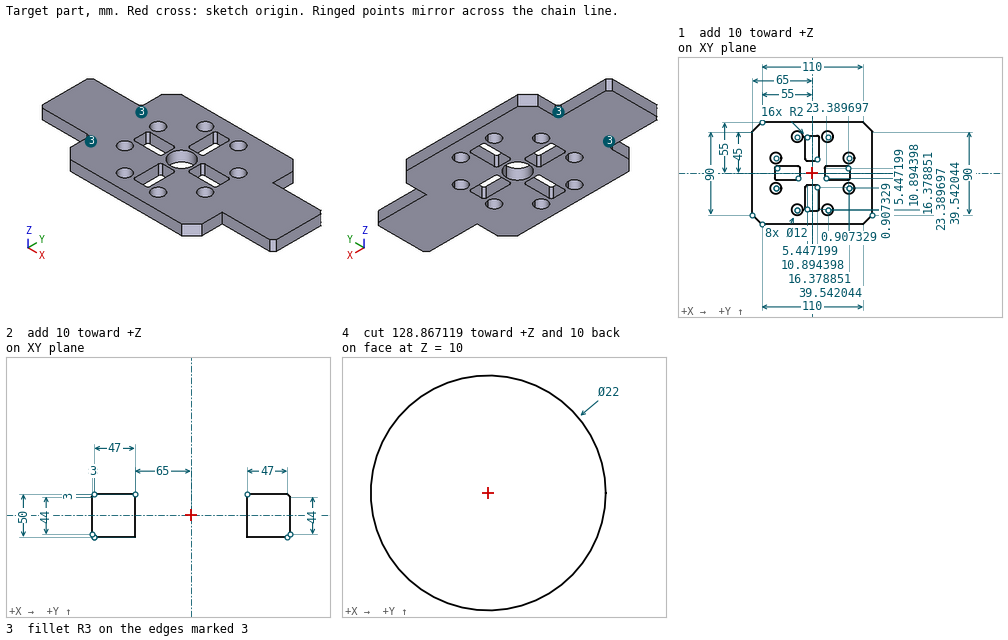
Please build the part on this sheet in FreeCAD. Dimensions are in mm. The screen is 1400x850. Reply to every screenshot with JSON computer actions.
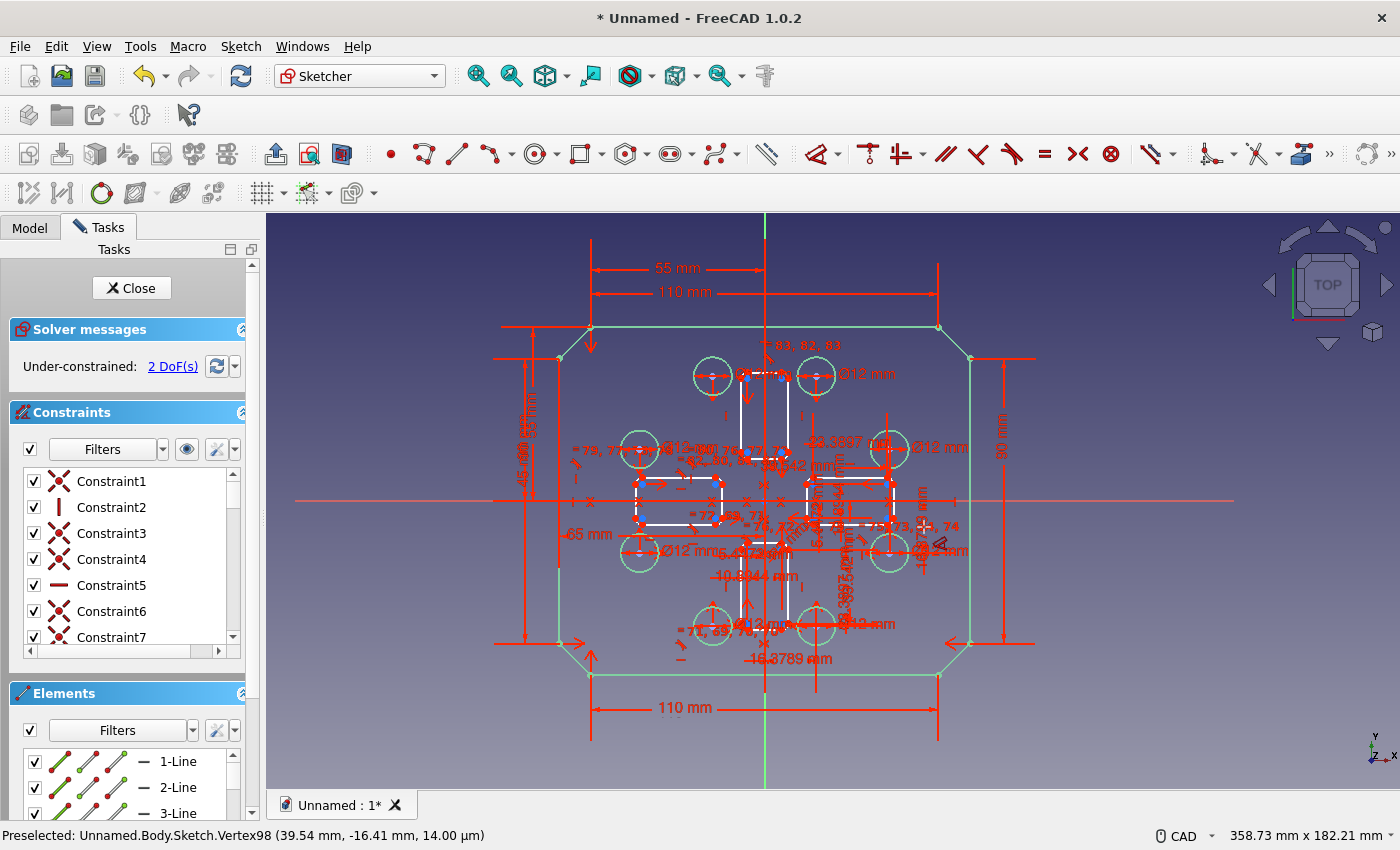
{"action": "scroll", "coordinate": [788, 624], "scroll_direction": "up", "scroll_amount": 14}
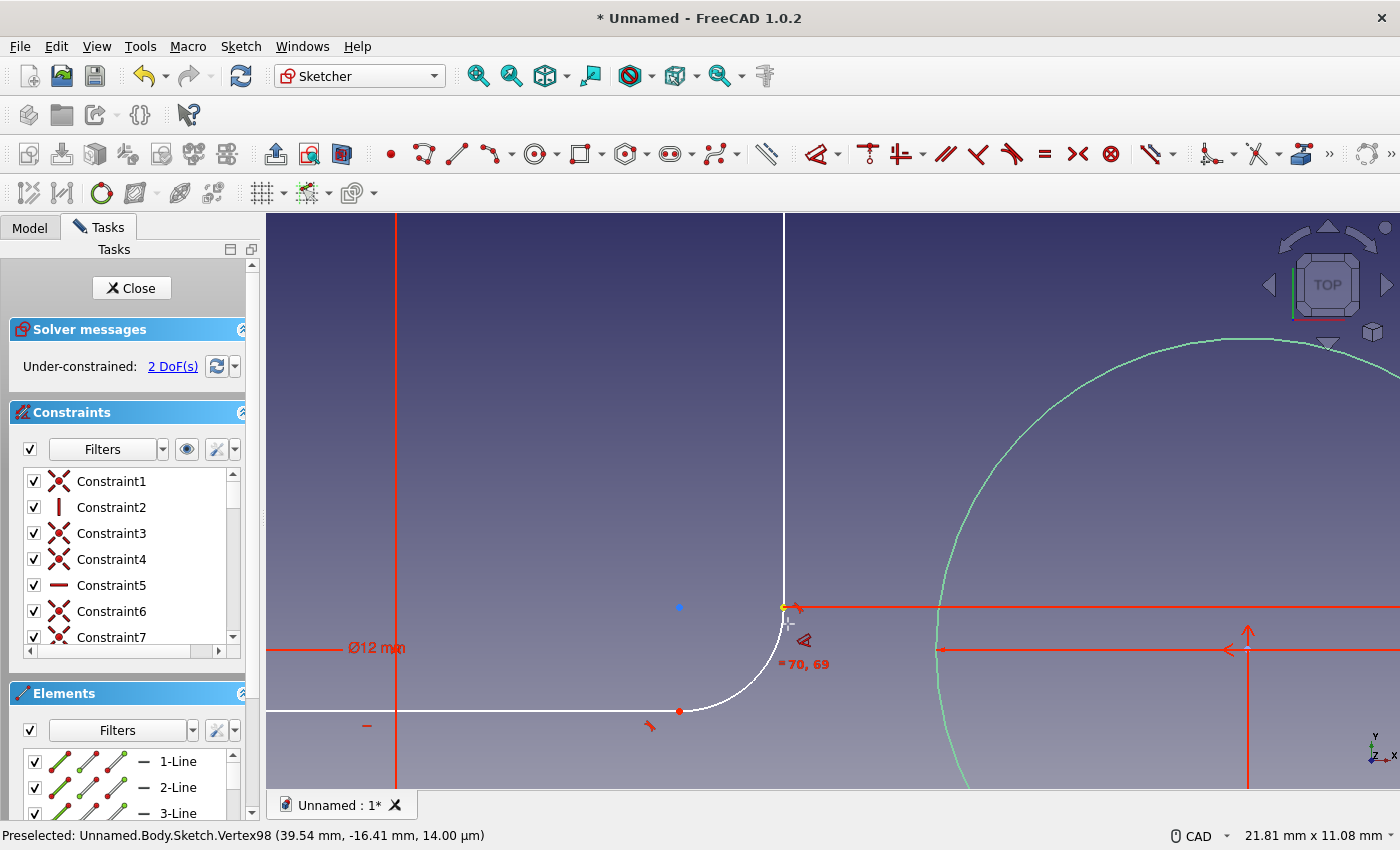
{"action": "left_click", "coordinate": [784, 607]}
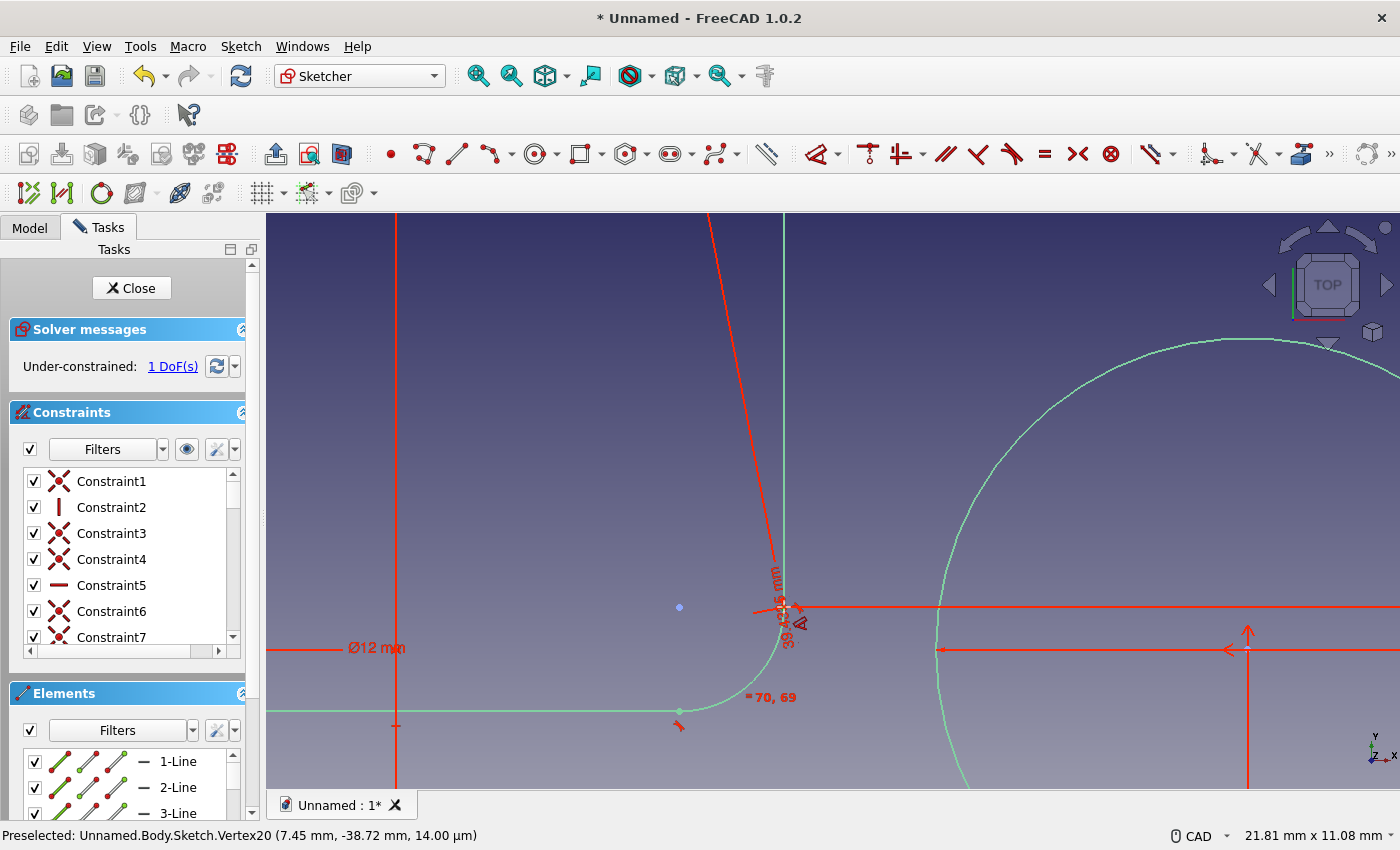
{"action": "scroll", "coordinate": [788, 624], "scroll_direction": "down", "scroll_amount": 14}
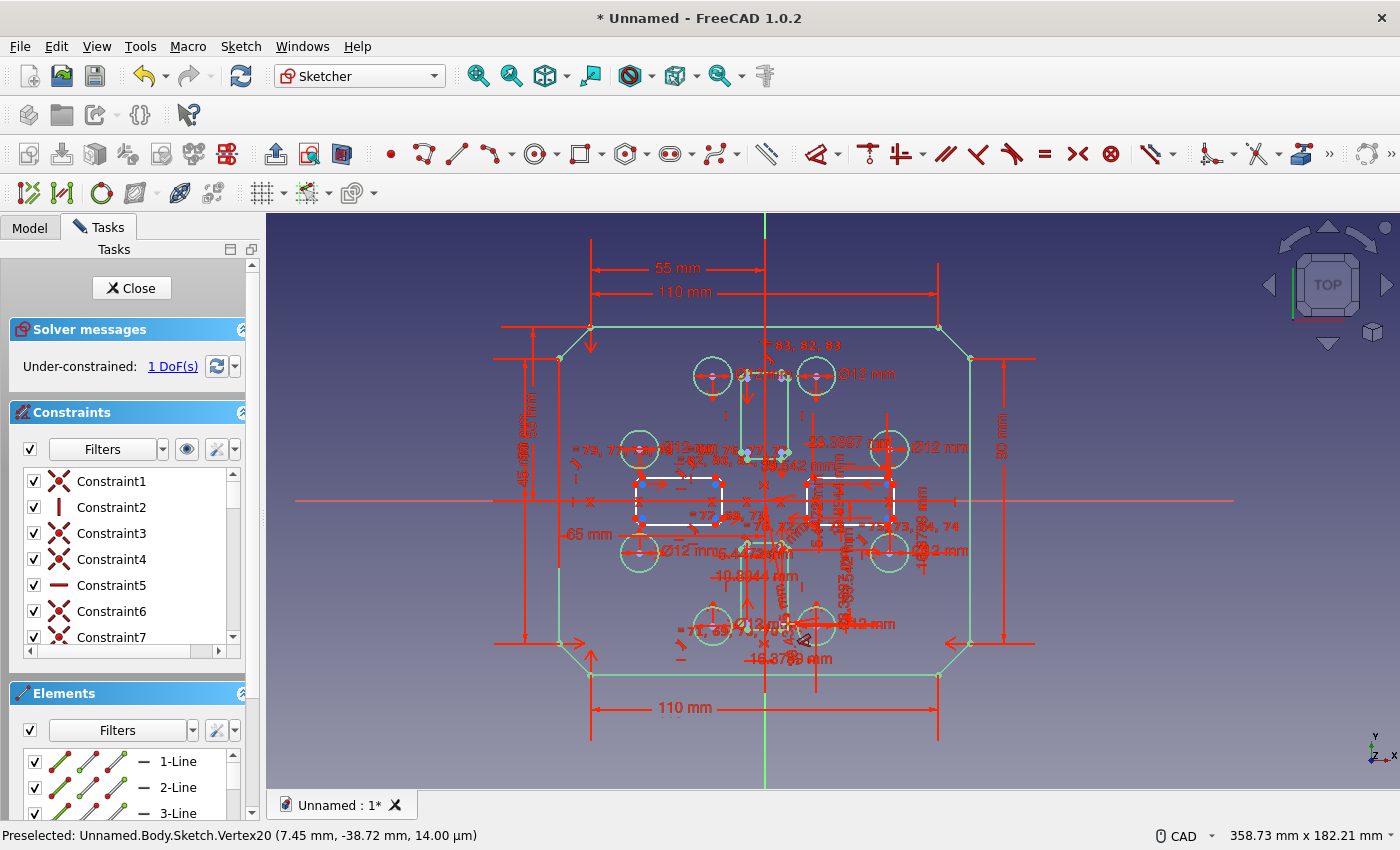
{"action": "scroll", "coordinate": [816, 626], "scroll_direction": "up", "scroll_amount": 14}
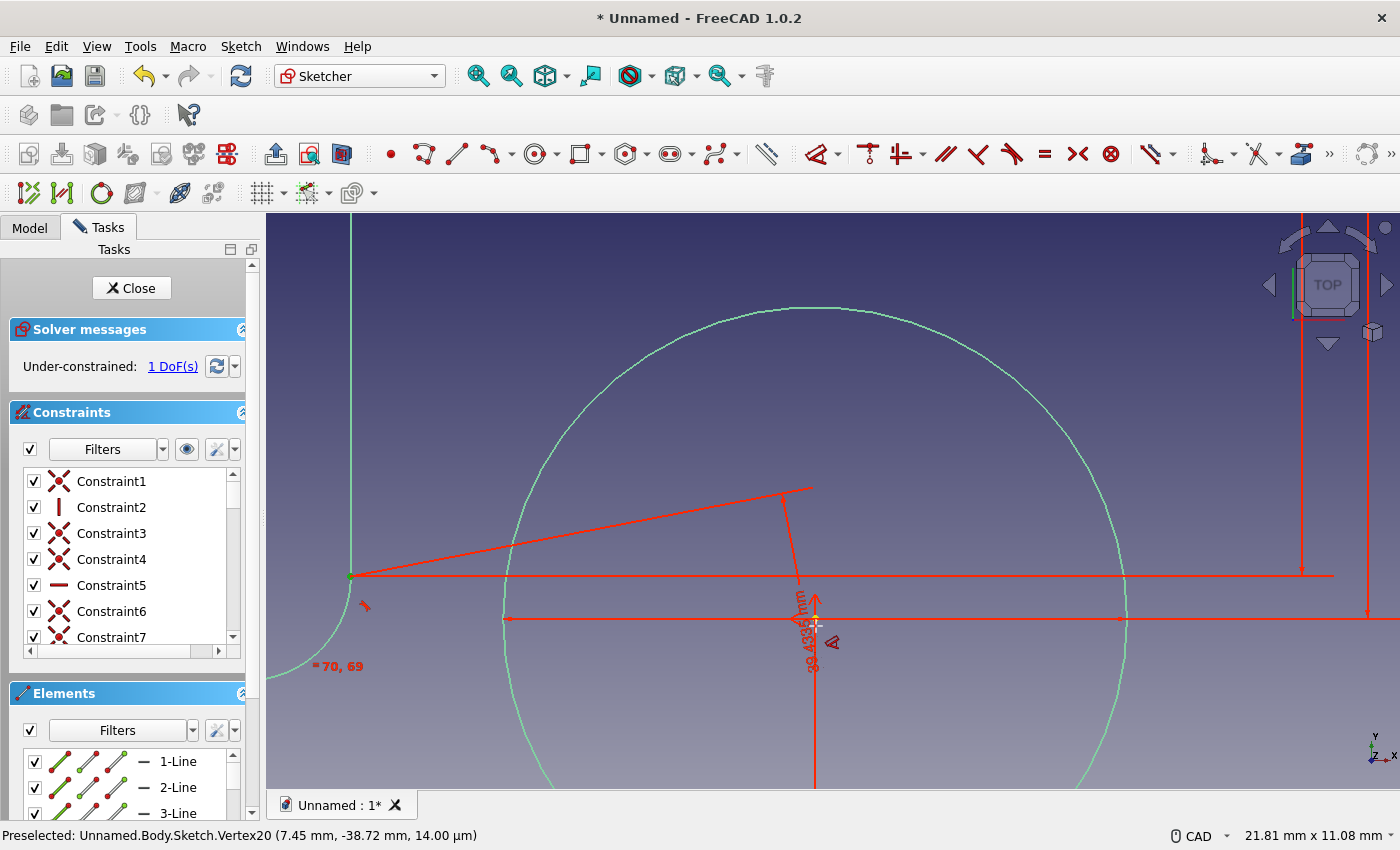
{"action": "left_click", "coordinate": [815, 619]}
{"action": "left_click", "coordinate": [849, 598]}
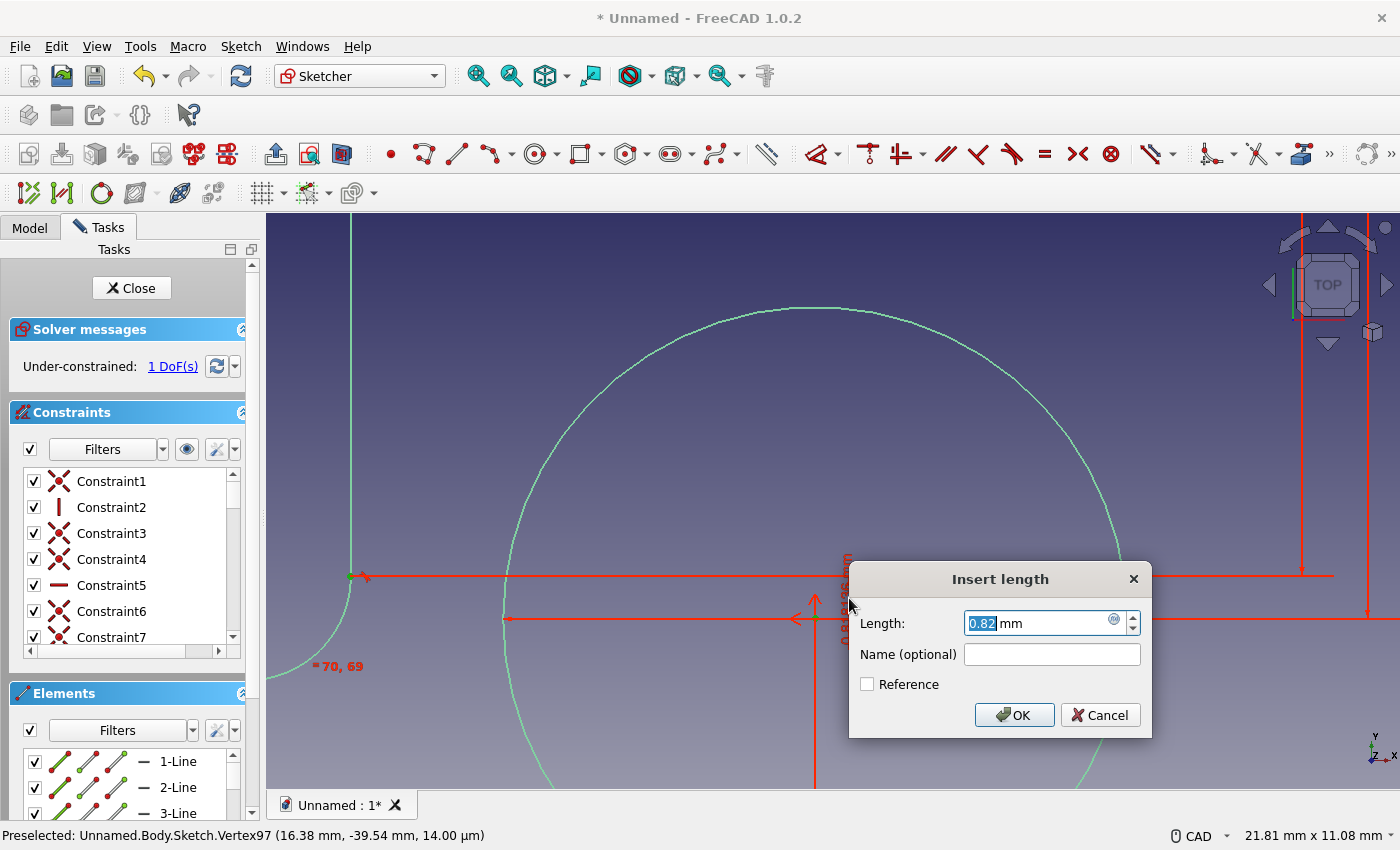
{"action": "type", "text": "0.907329"}
{"action": "key", "text": "Return"}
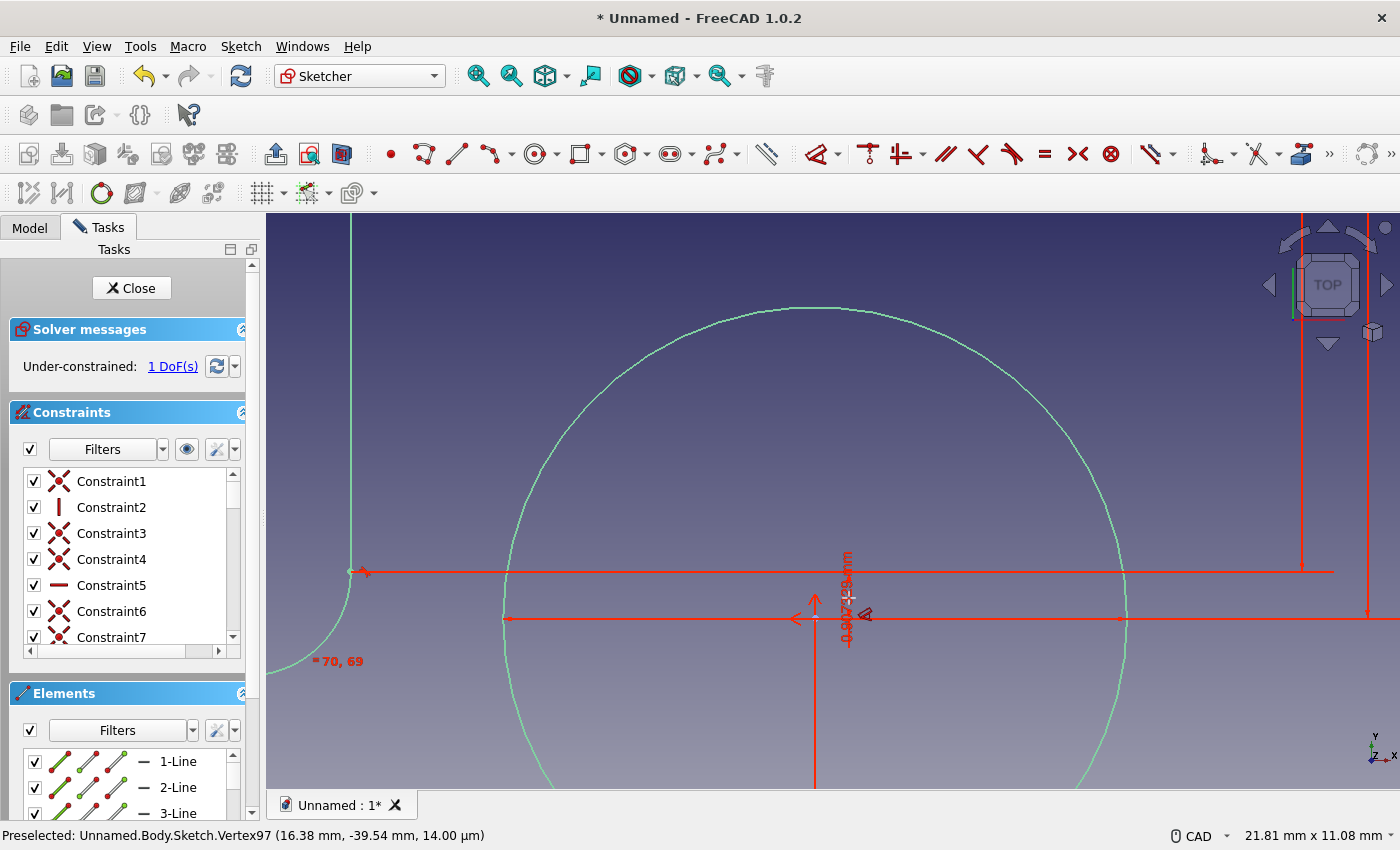
{"action": "scroll", "coordinate": [816, 626], "scroll_direction": "down", "scroll_amount": 14}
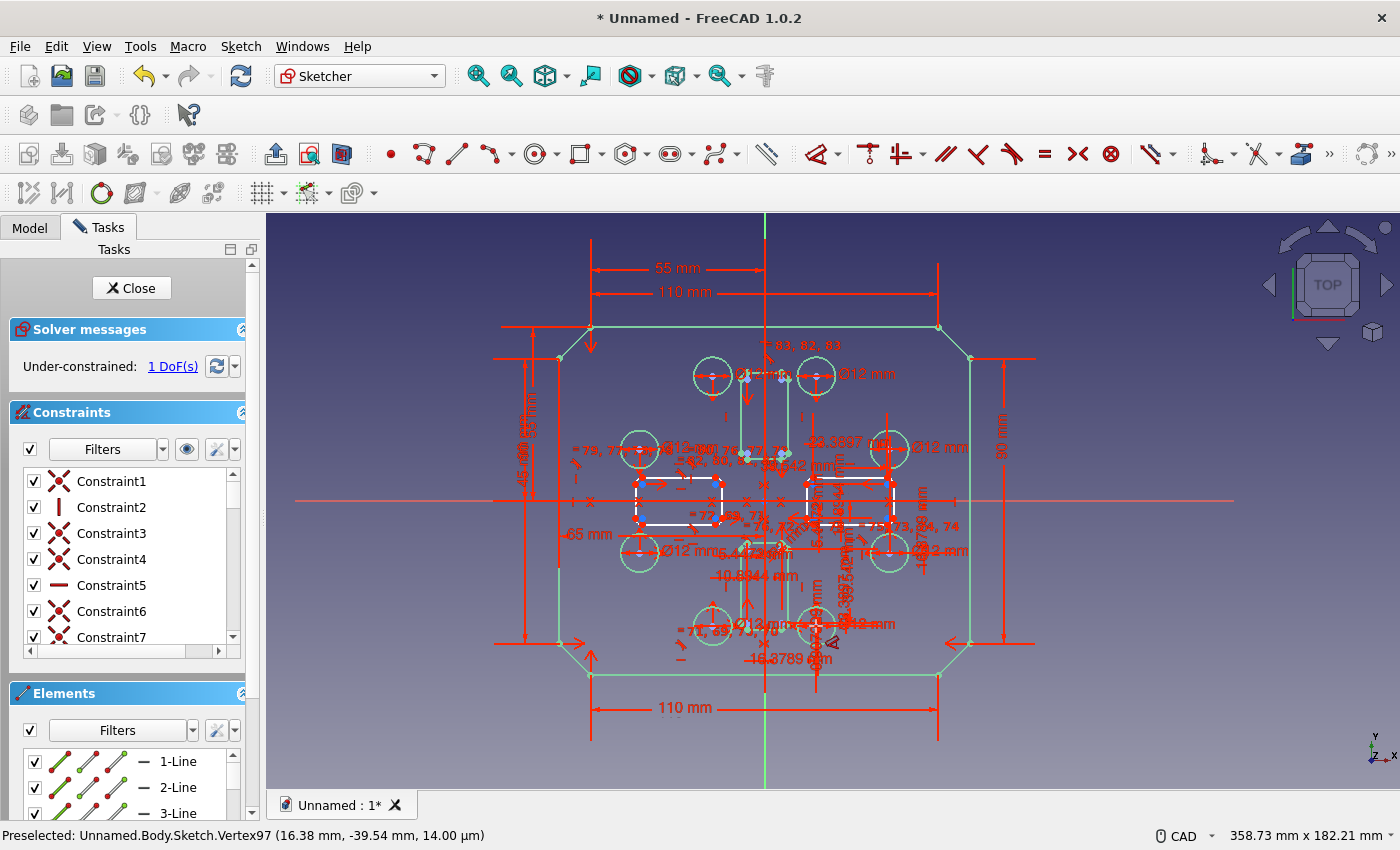
{"action": "scroll", "coordinate": [887, 525], "scroll_direction": "up", "scroll_amount": 14}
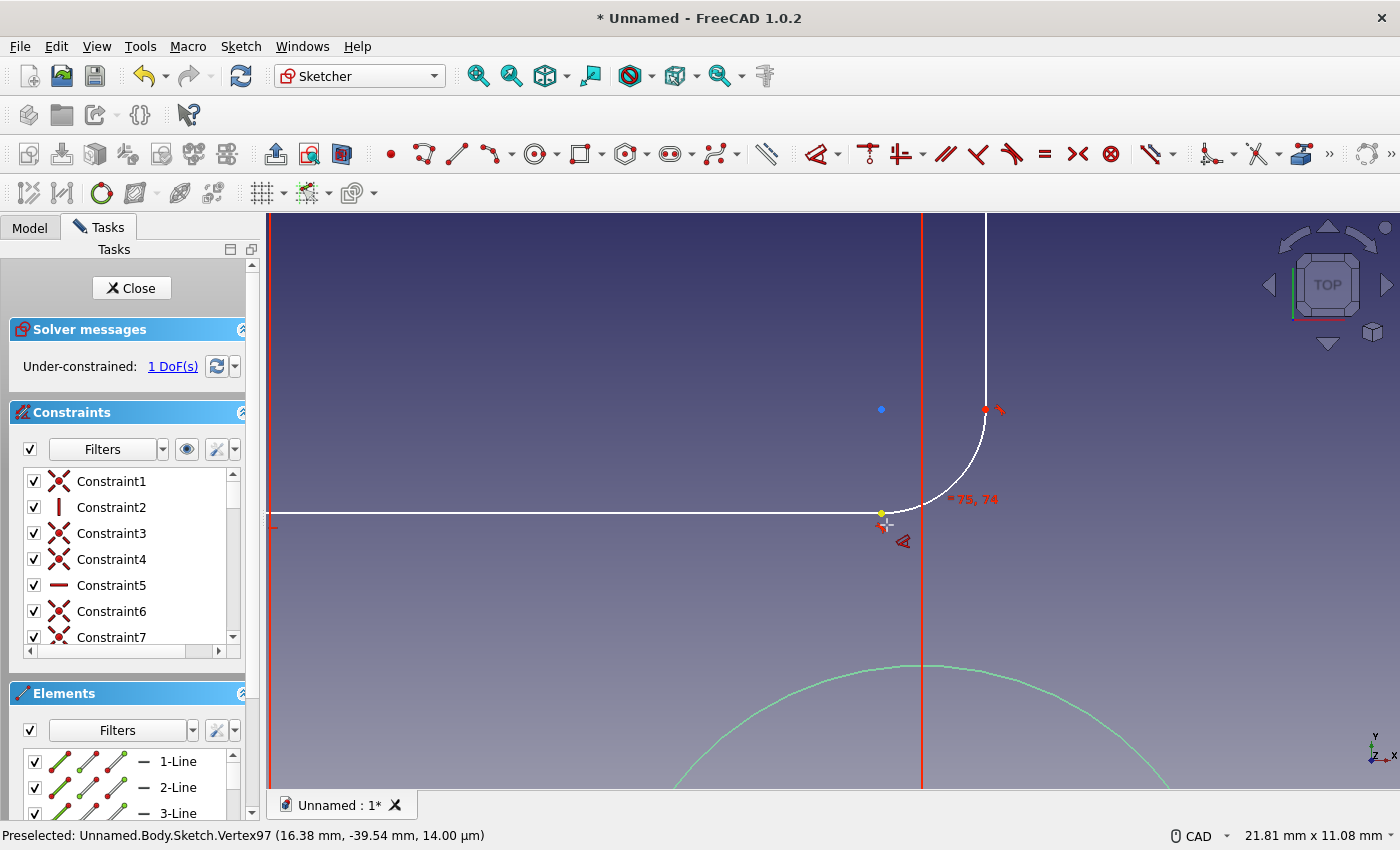
{"action": "left_click", "coordinate": [882, 513]}